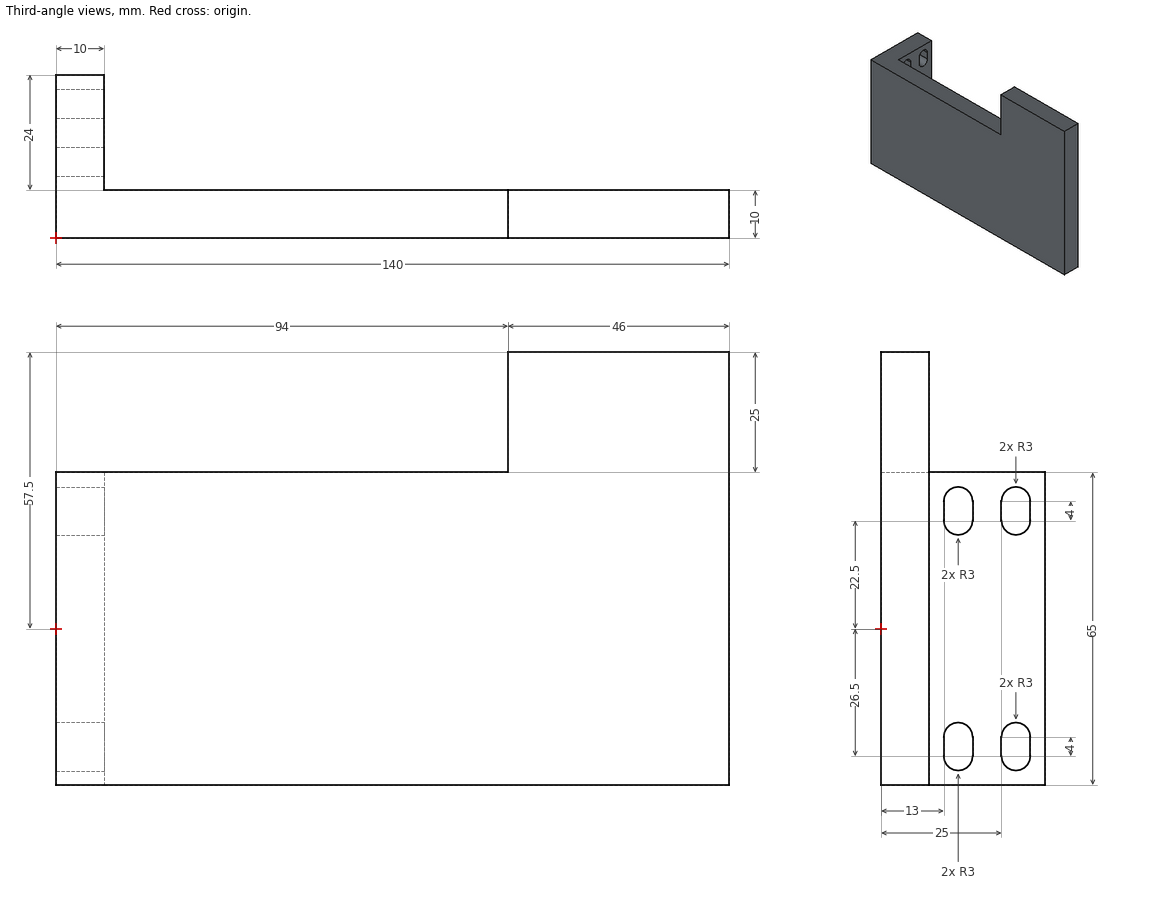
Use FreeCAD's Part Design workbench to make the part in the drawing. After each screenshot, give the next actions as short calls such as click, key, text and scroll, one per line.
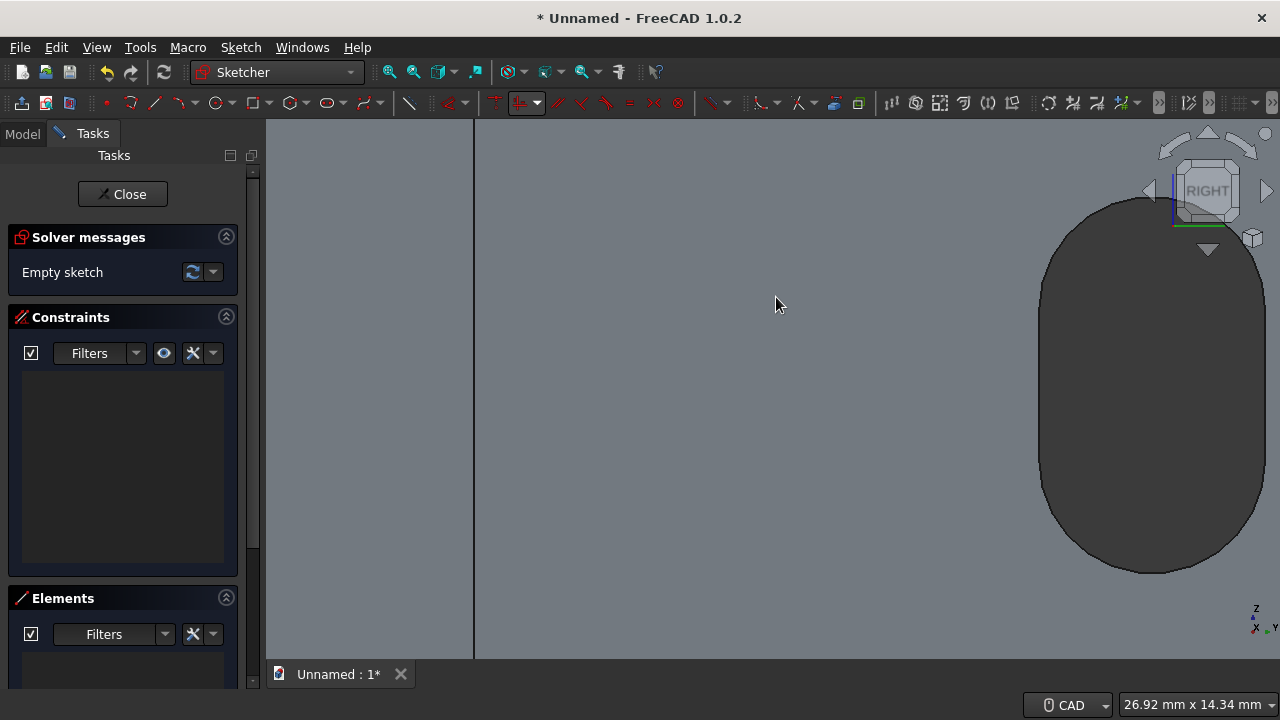
click(328, 104)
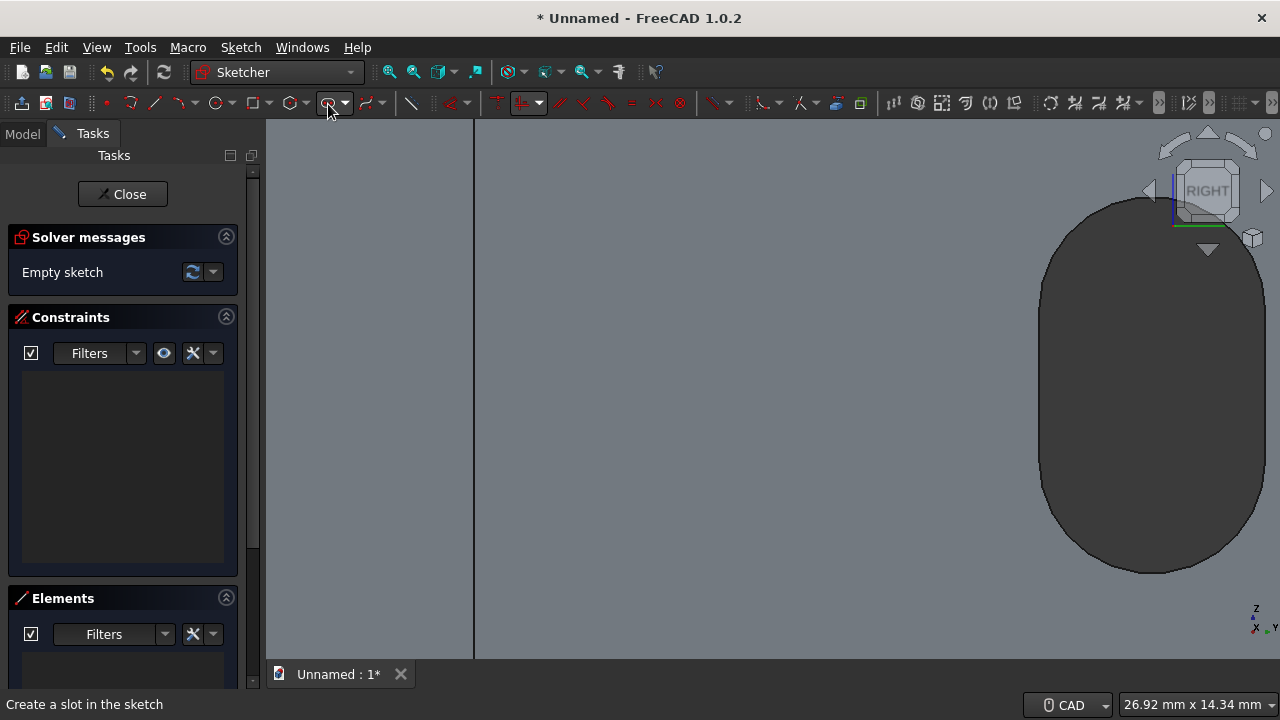
click(700, 460)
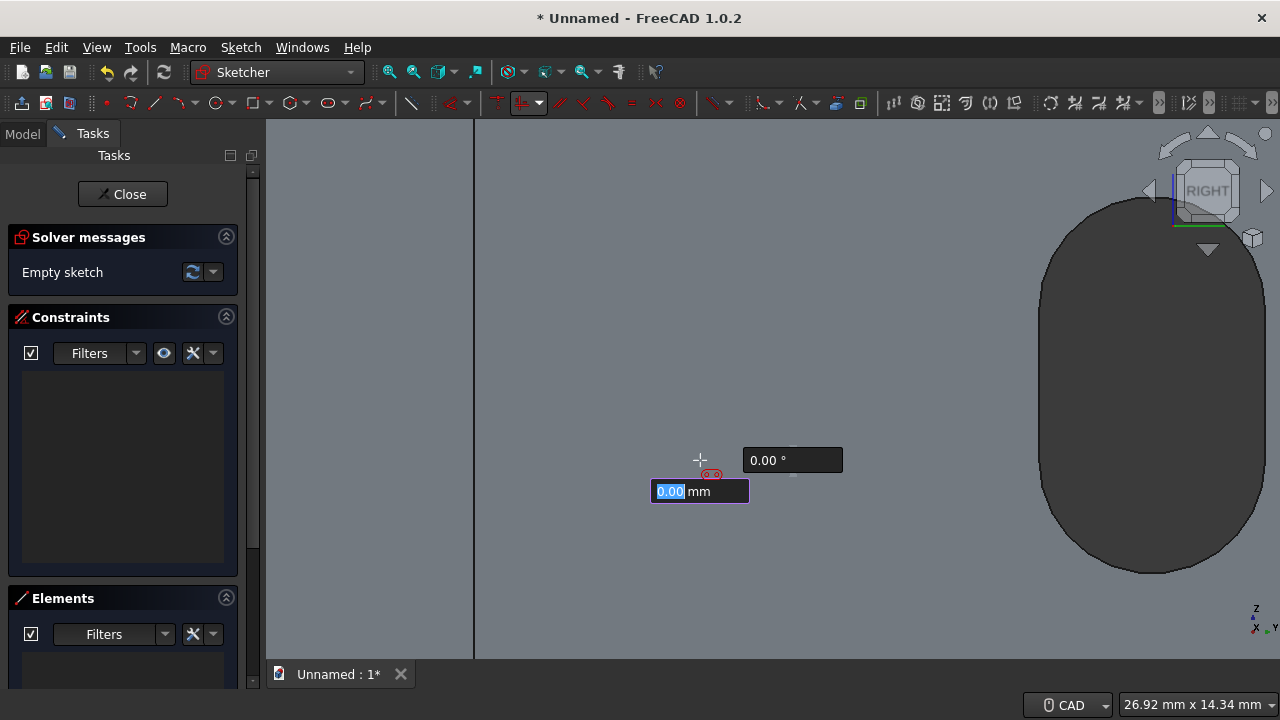
click(700, 310)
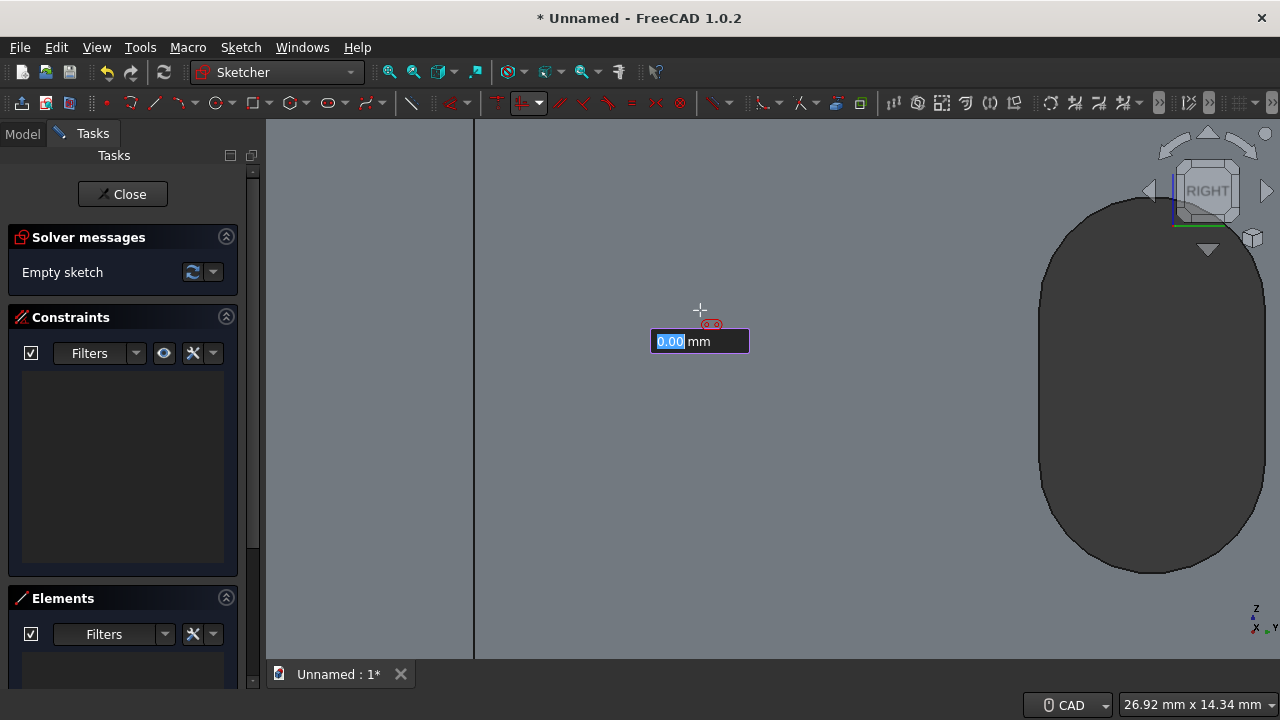
click(587, 385)
key(Escape)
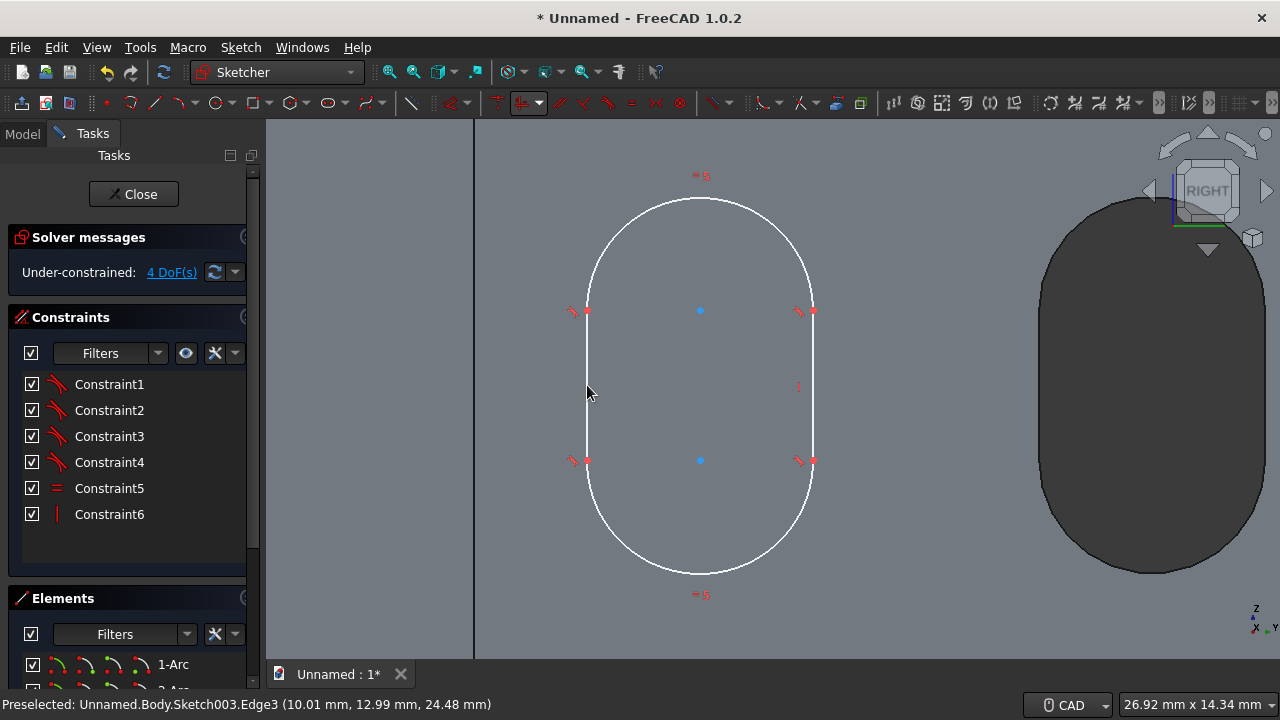
key(d)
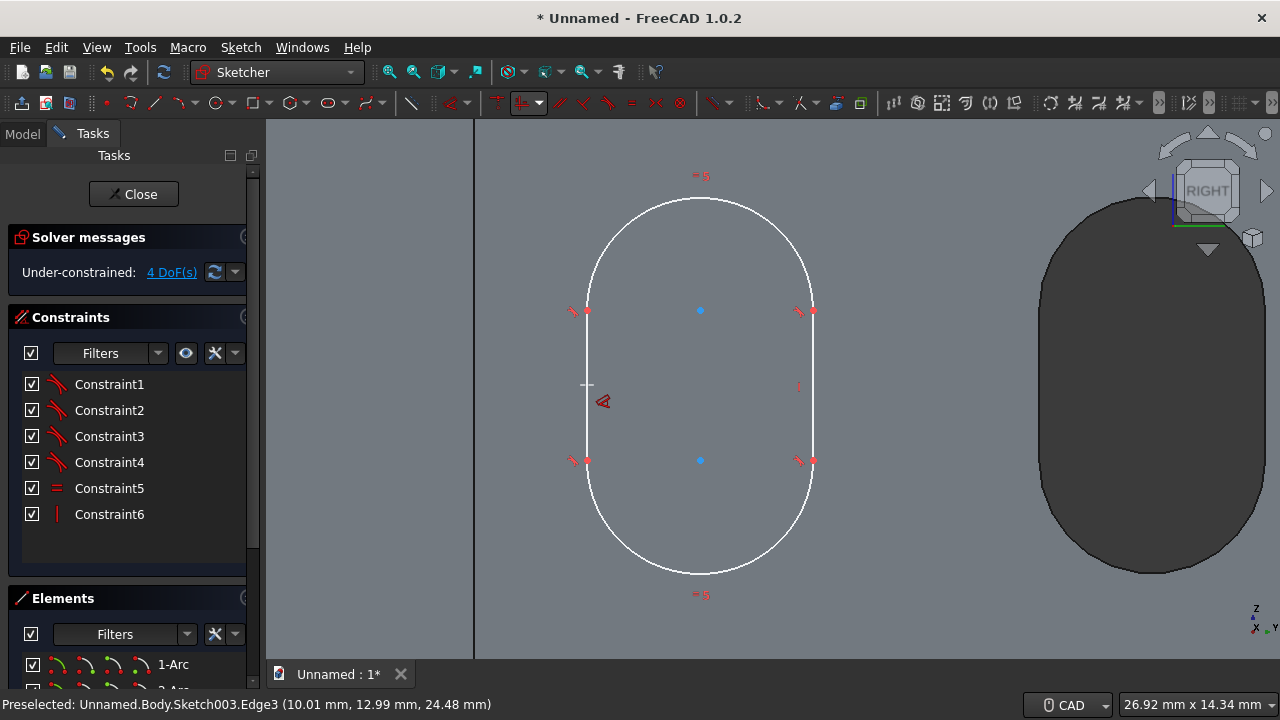
click(634, 552)
click(615, 578)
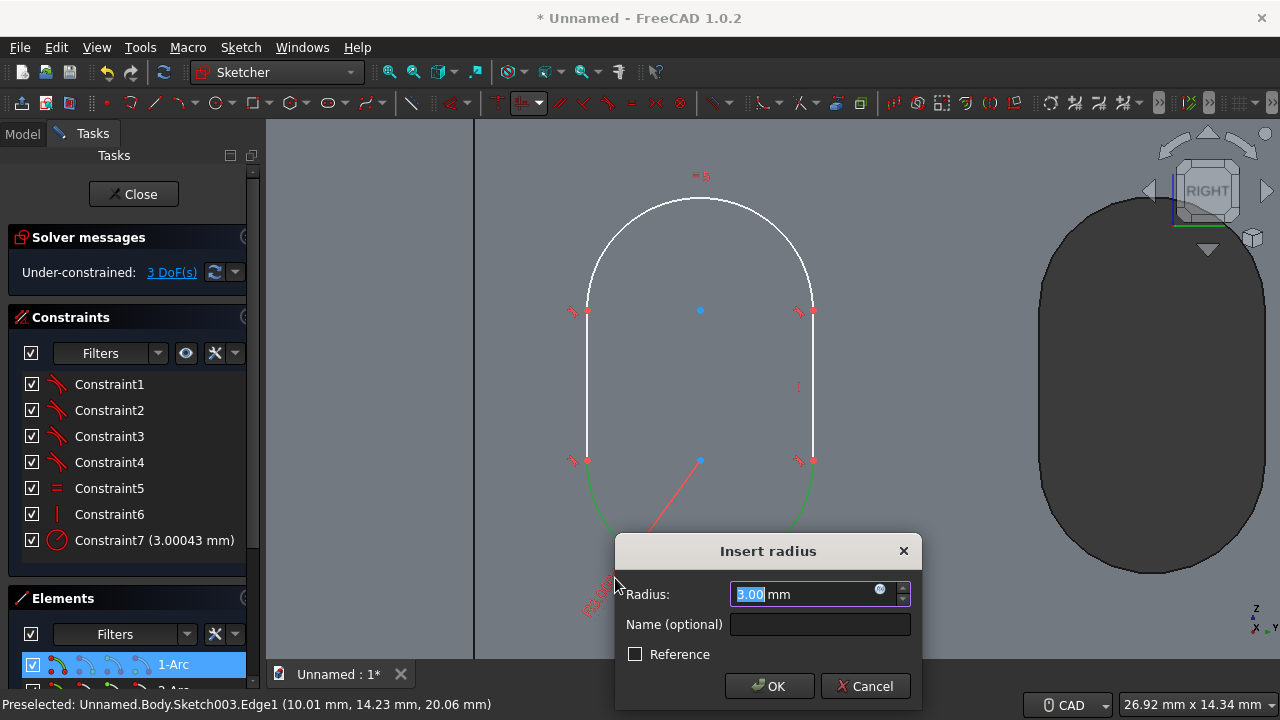
text(3)
key(Return)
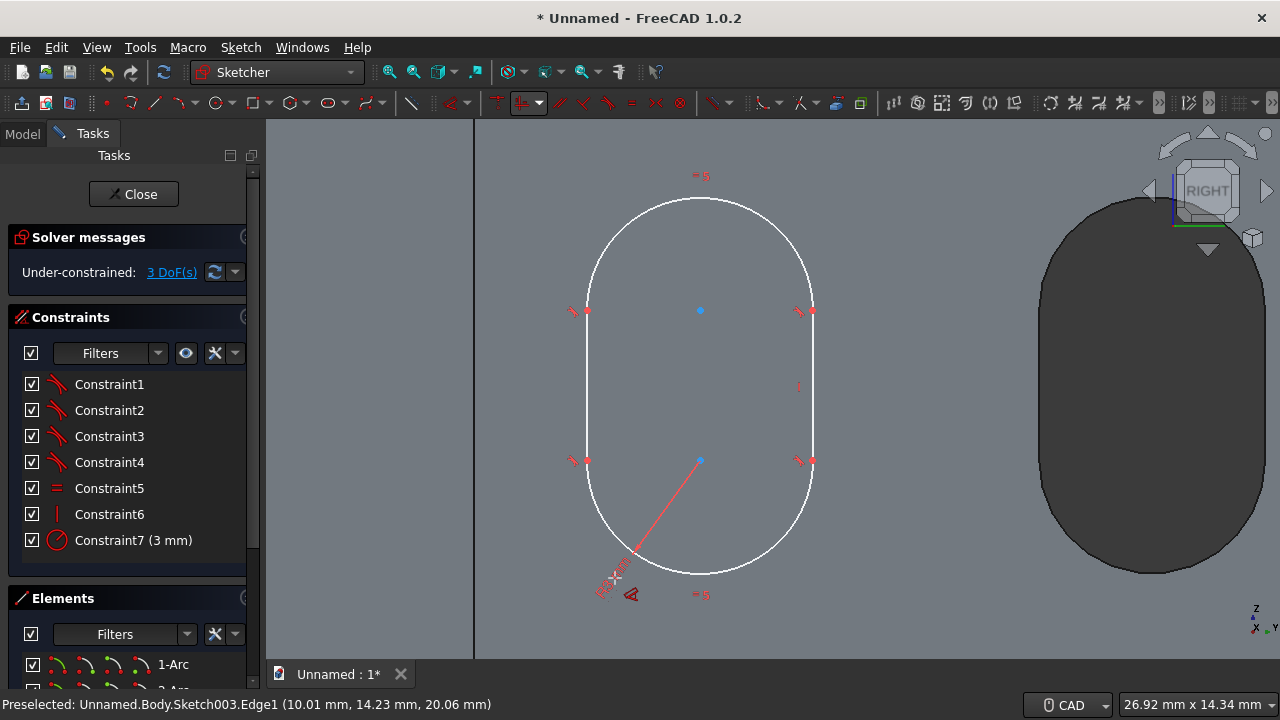
click(587, 416)
click(553, 386)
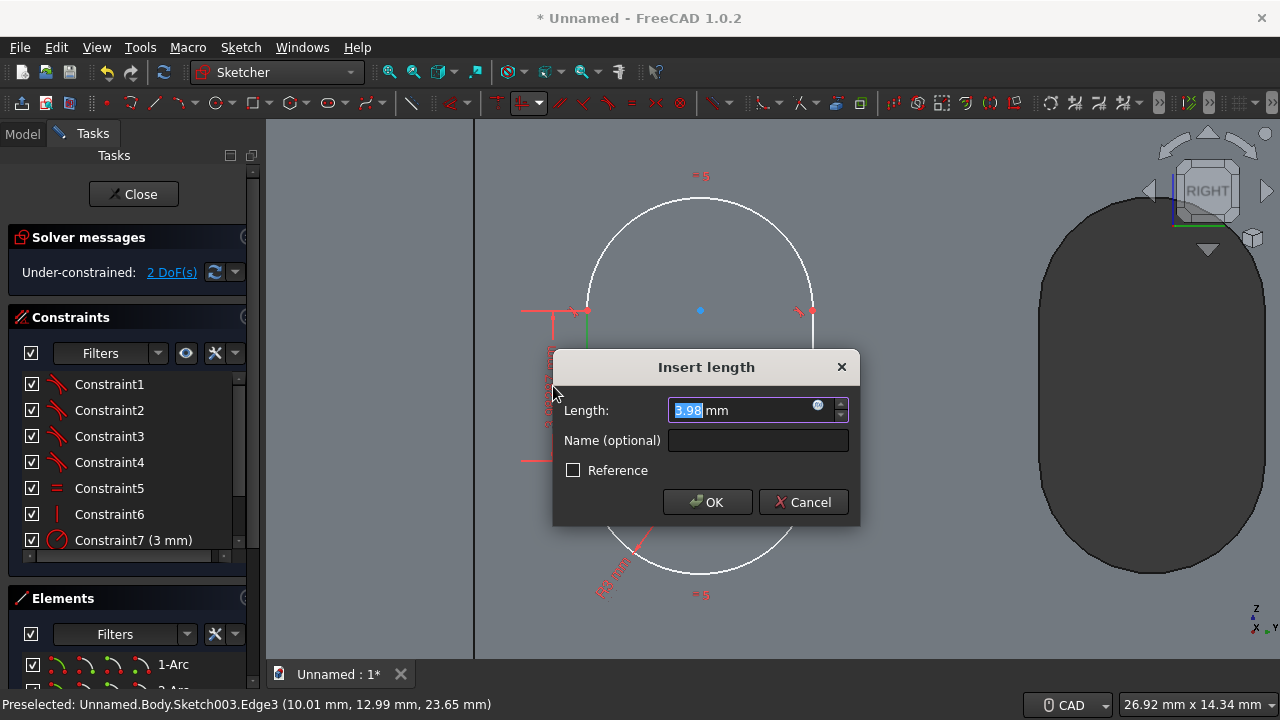
text(4)
key(Return)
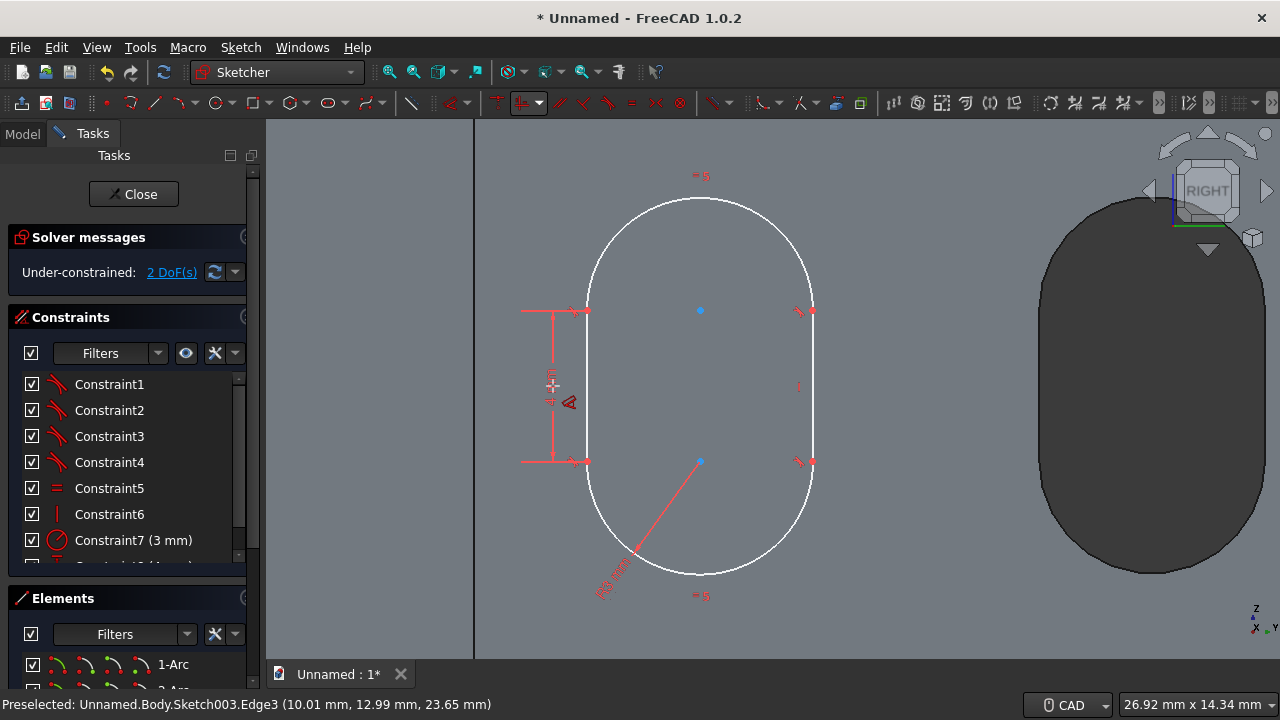
click(587, 462)
click(441, 428)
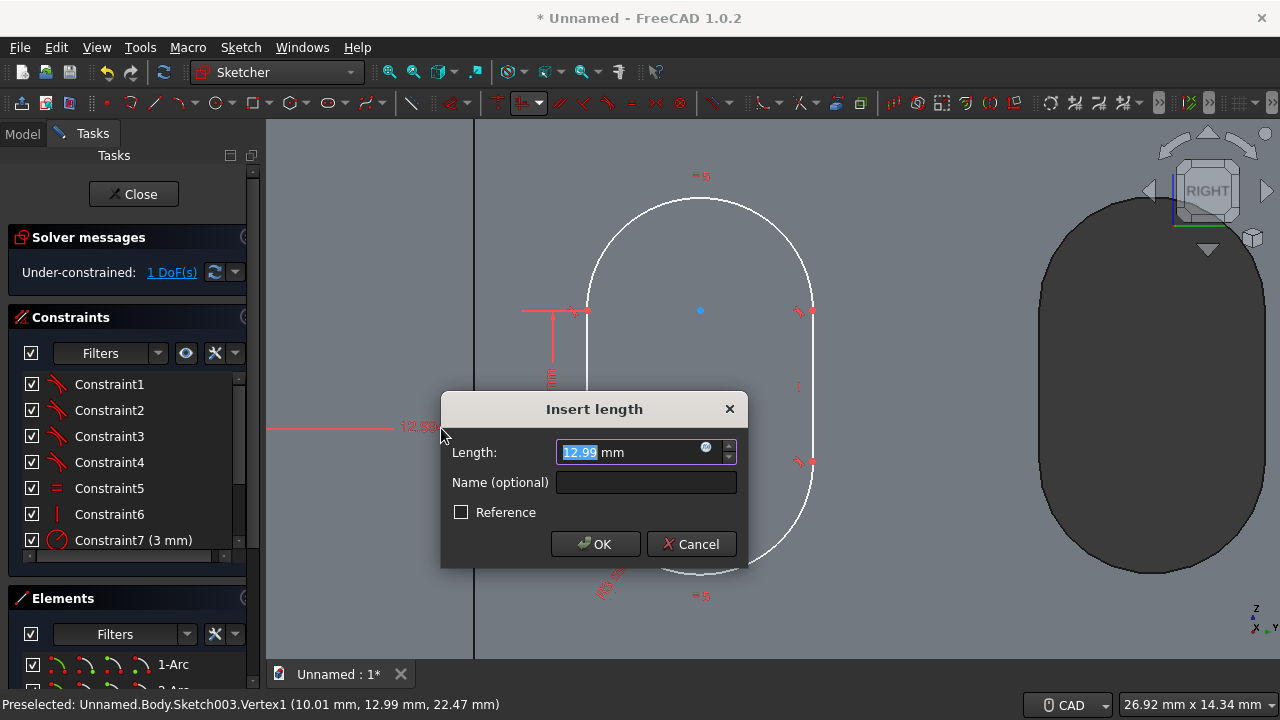
text(13)
key(Return)